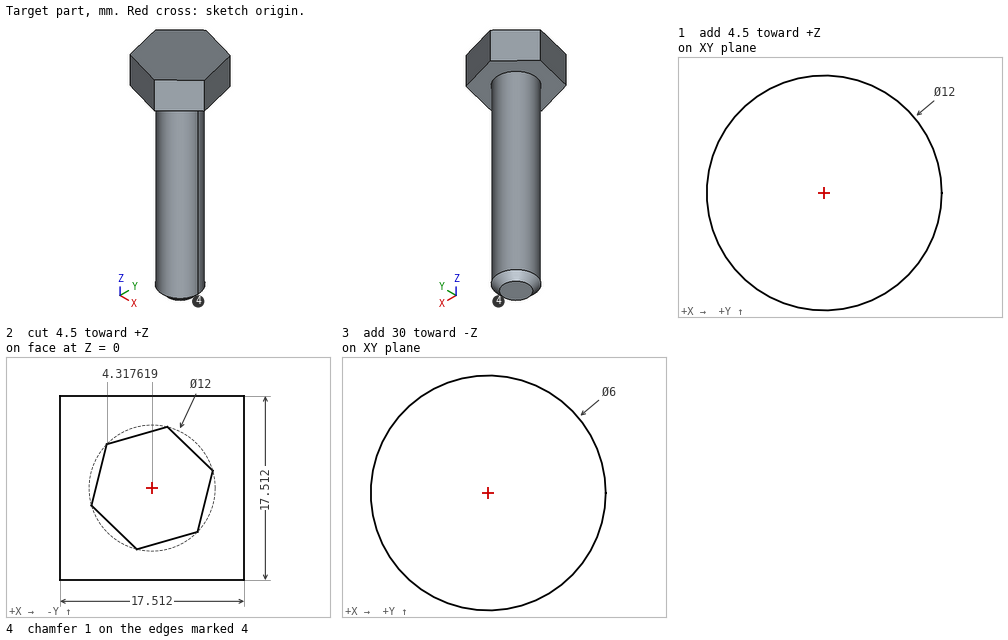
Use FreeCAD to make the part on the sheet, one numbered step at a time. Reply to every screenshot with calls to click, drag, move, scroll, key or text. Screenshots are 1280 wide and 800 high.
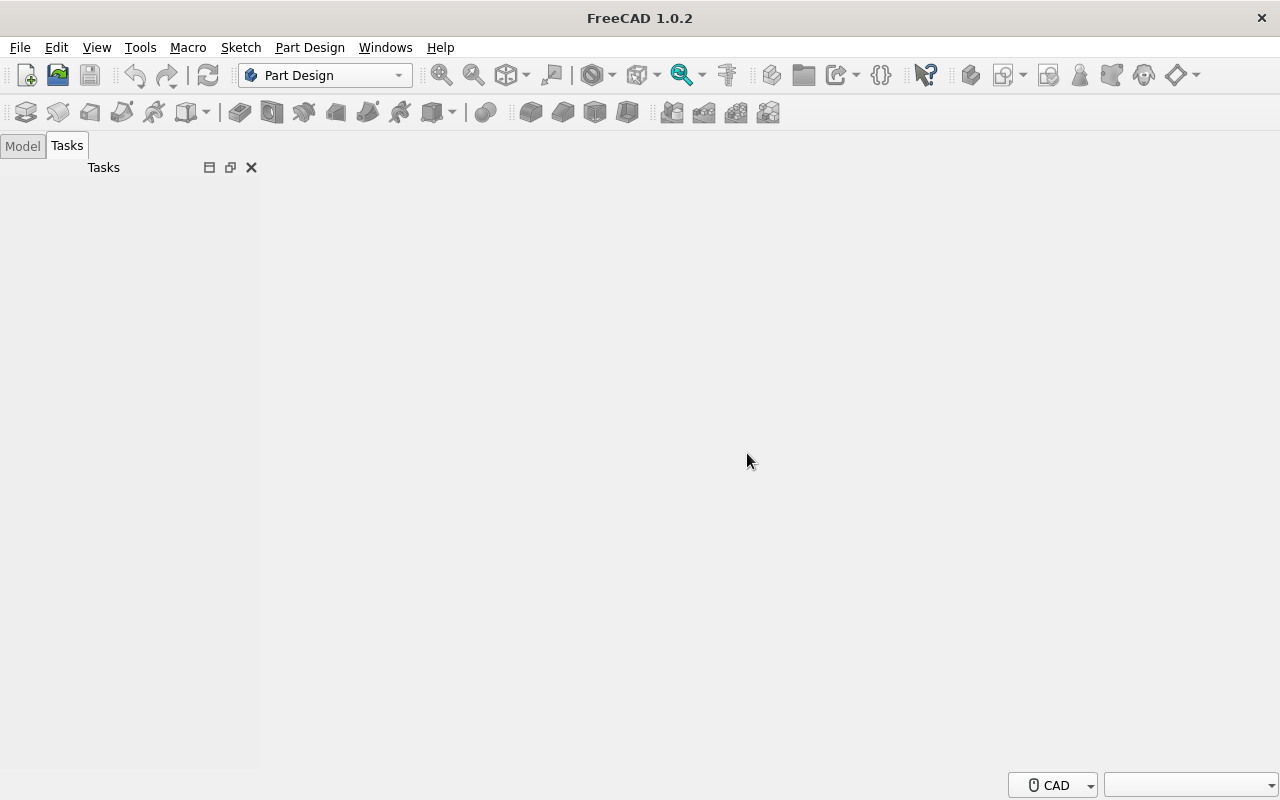
key(ctrl+n)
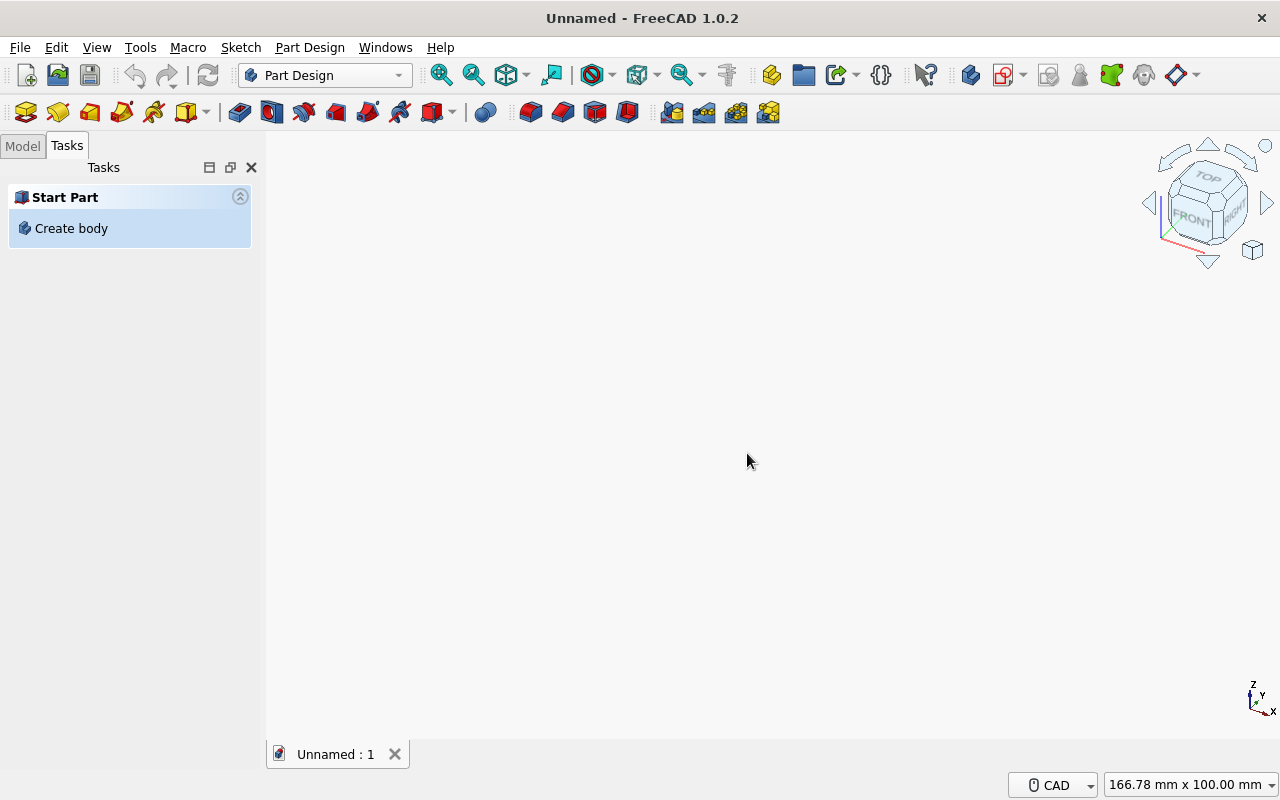
click(1004, 76)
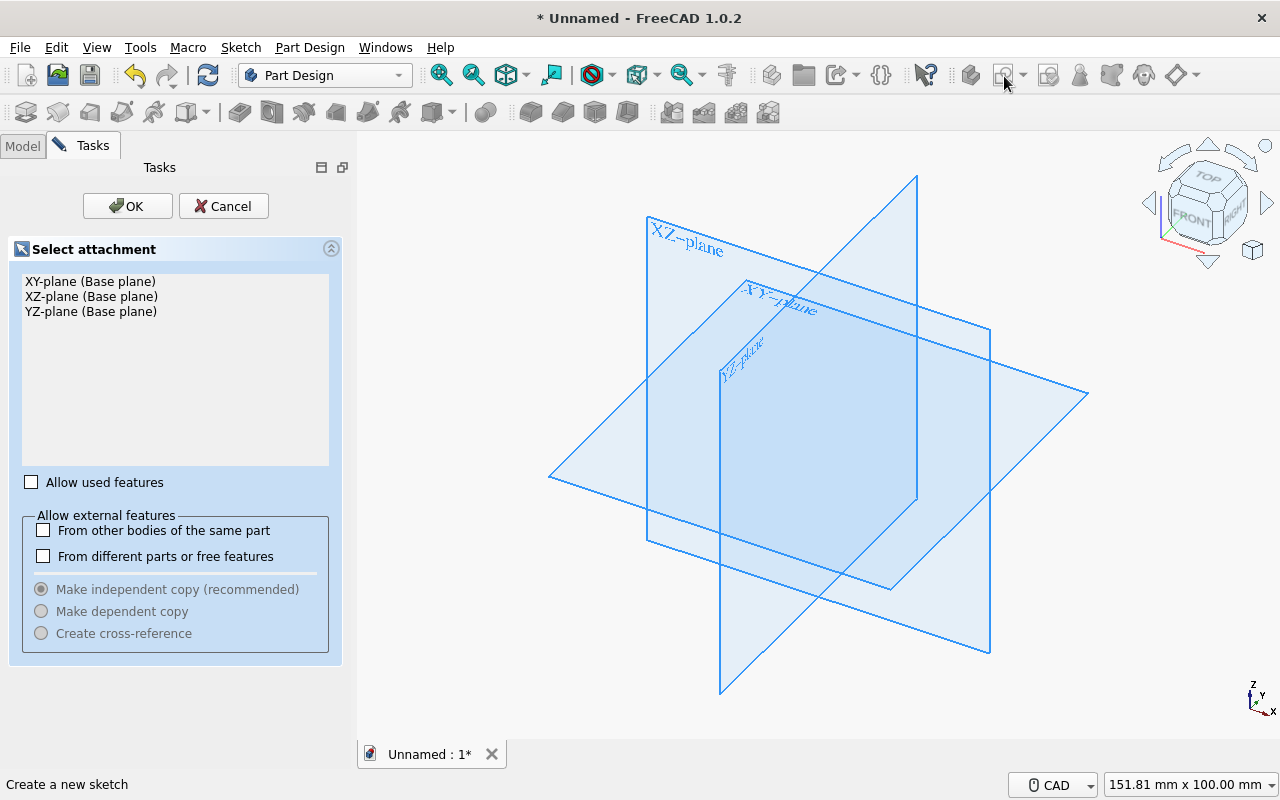
click(82, 282)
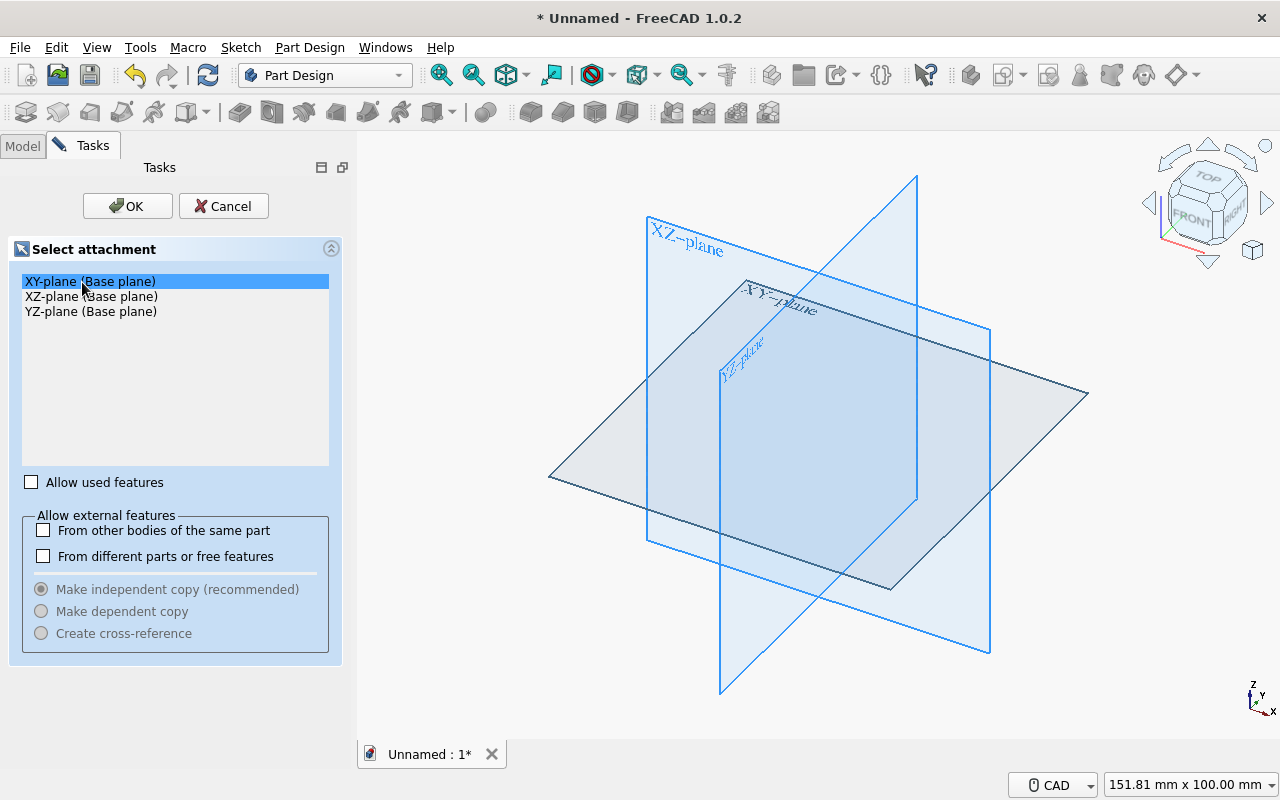
click(128, 206)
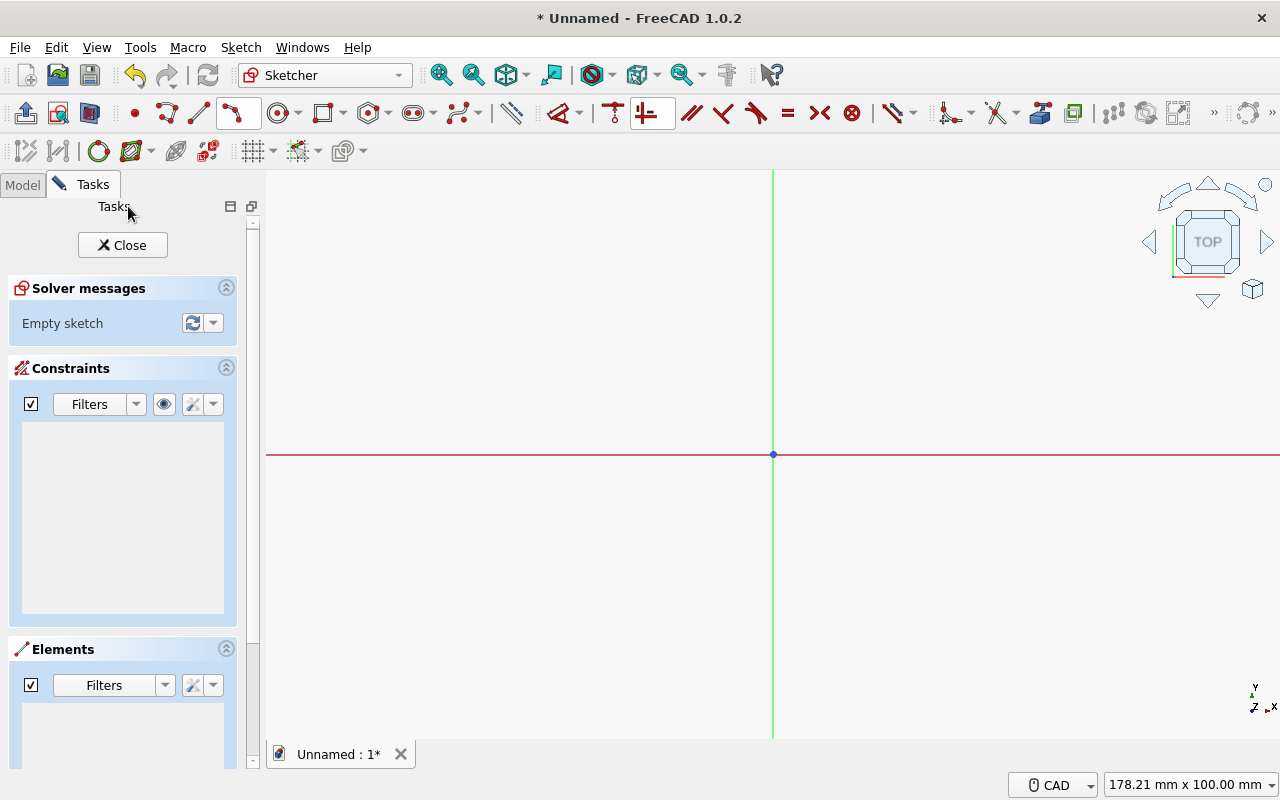
scroll(790, 454, up, 8)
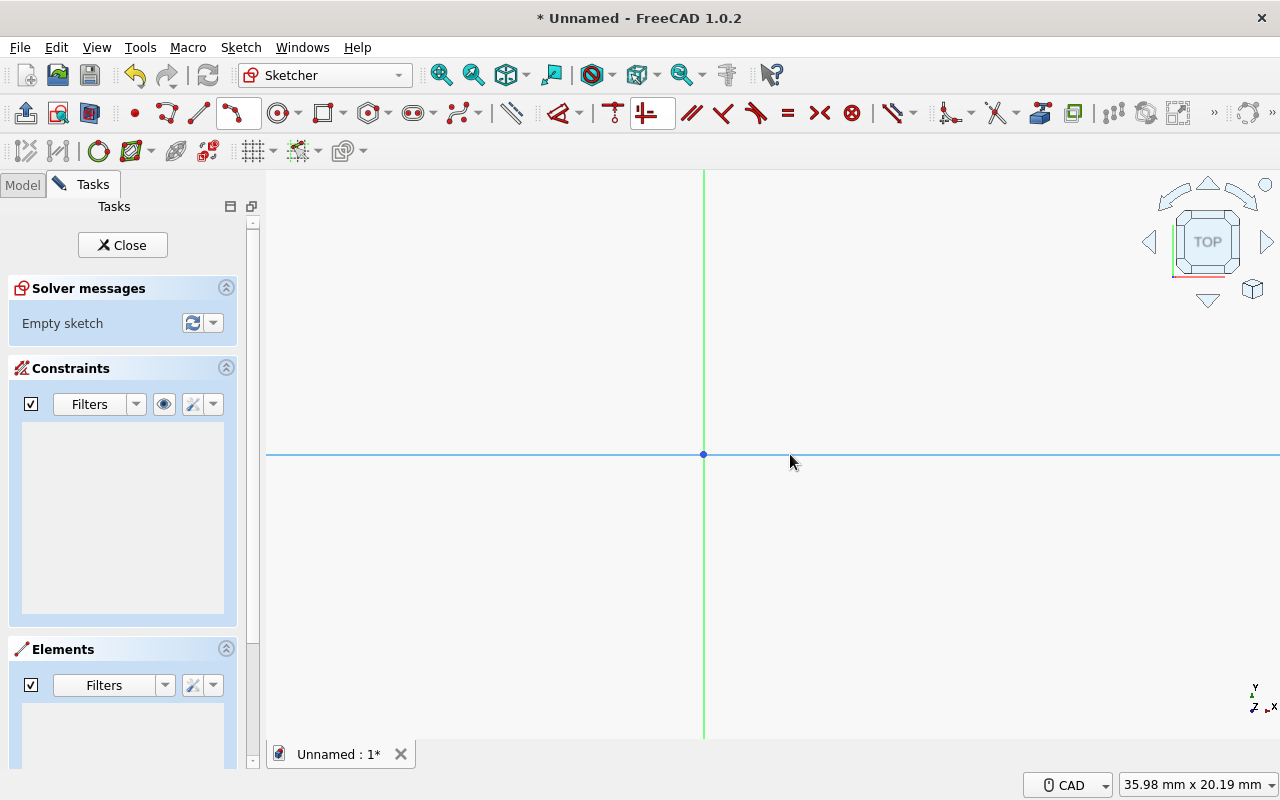
click(278, 114)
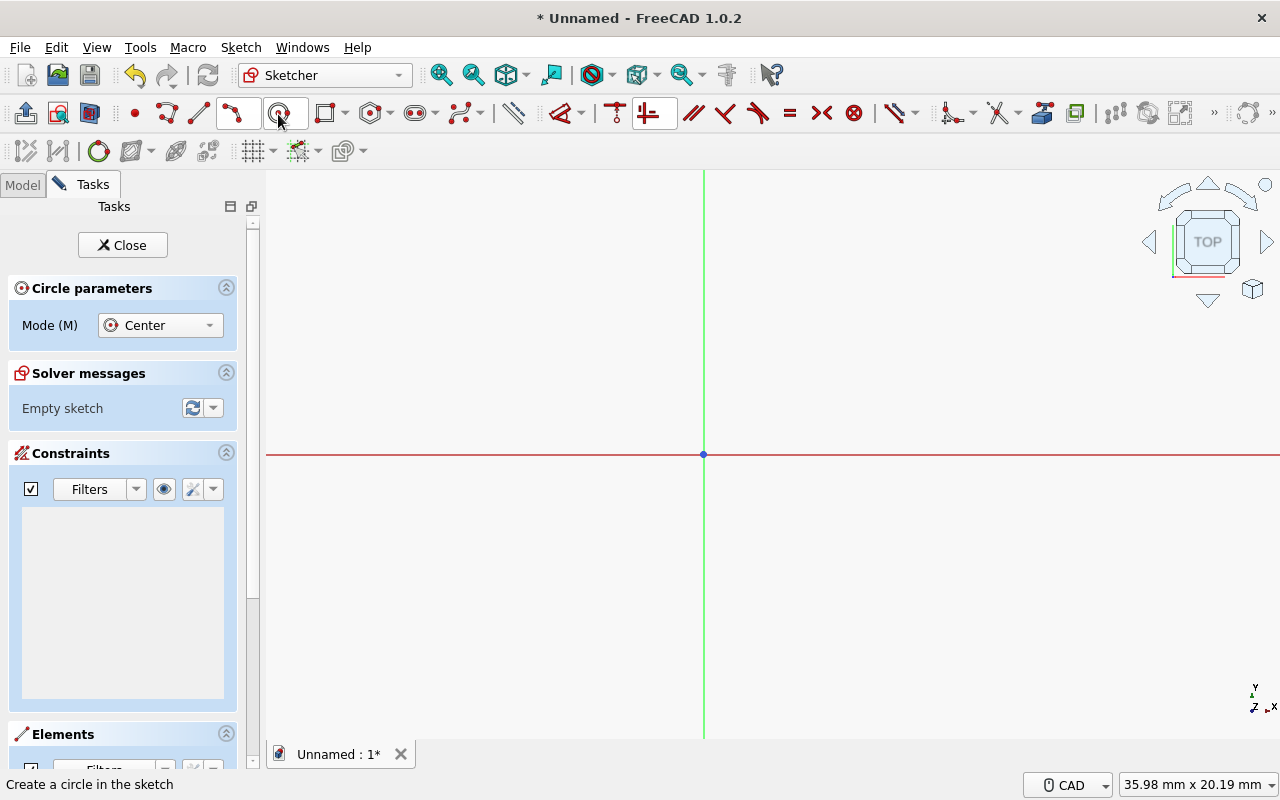
click(704, 454)
click(823, 335)
key(Escape)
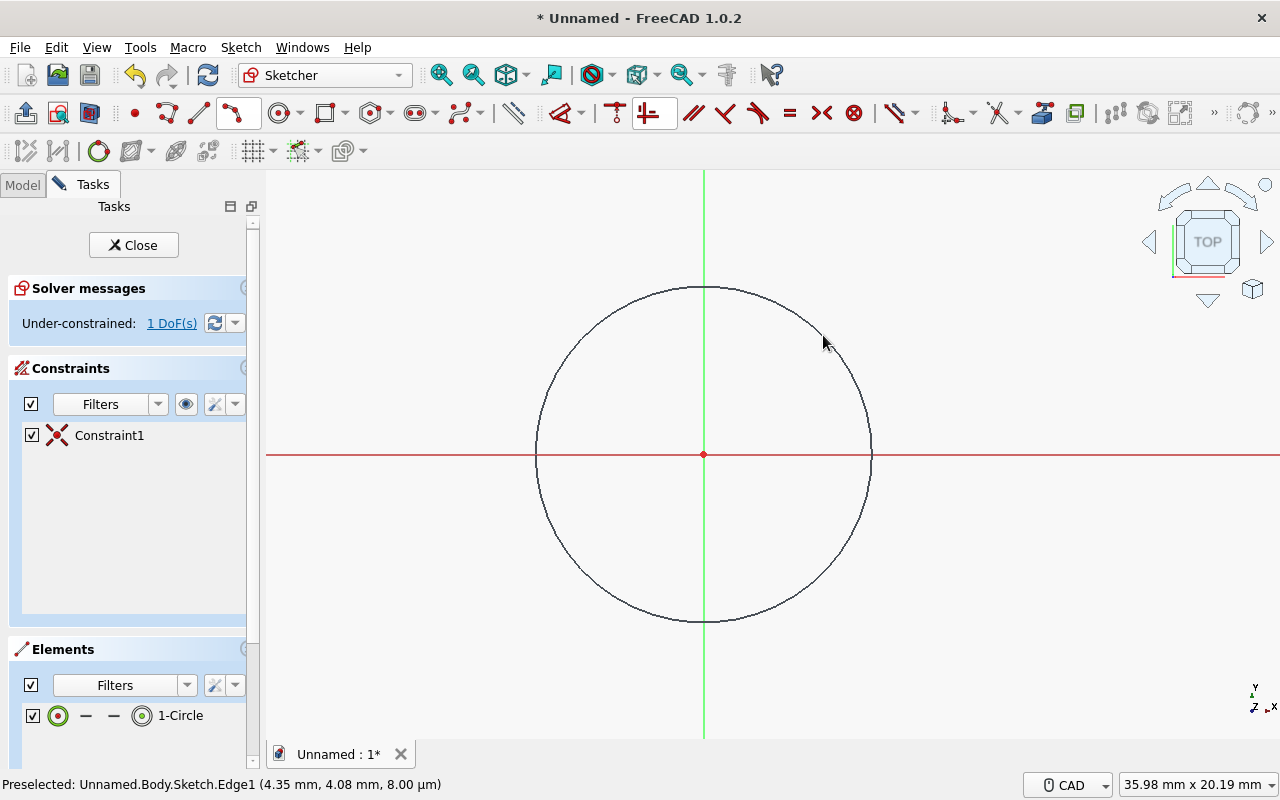
click(822, 335)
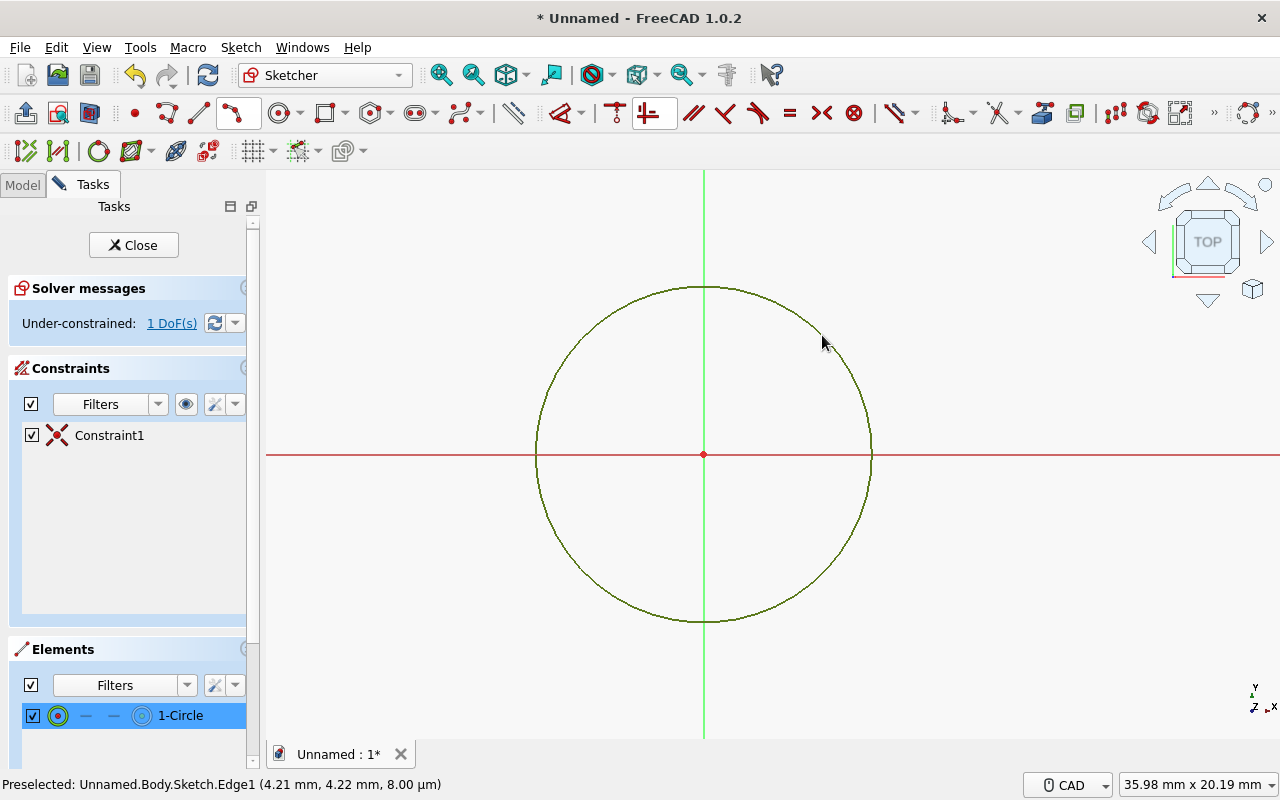
key(k)
key(o)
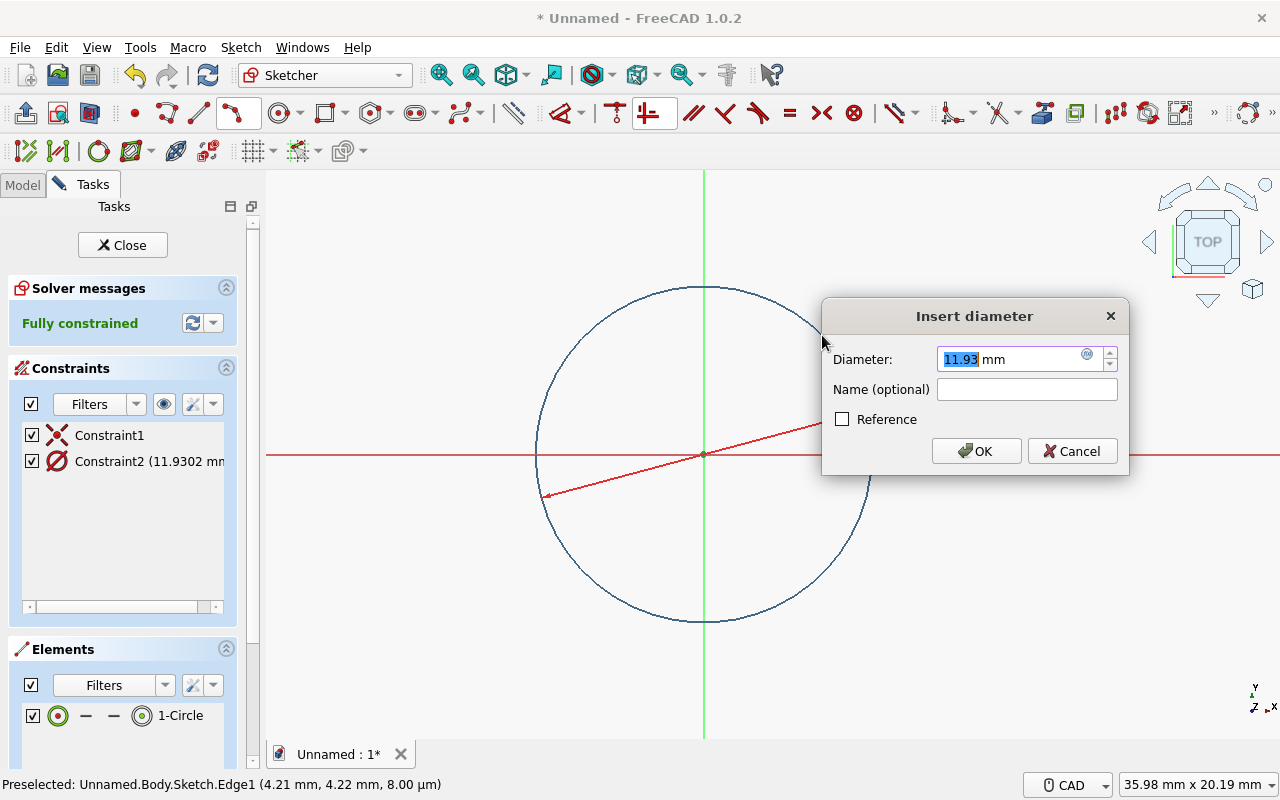
text(12)
key(Return)